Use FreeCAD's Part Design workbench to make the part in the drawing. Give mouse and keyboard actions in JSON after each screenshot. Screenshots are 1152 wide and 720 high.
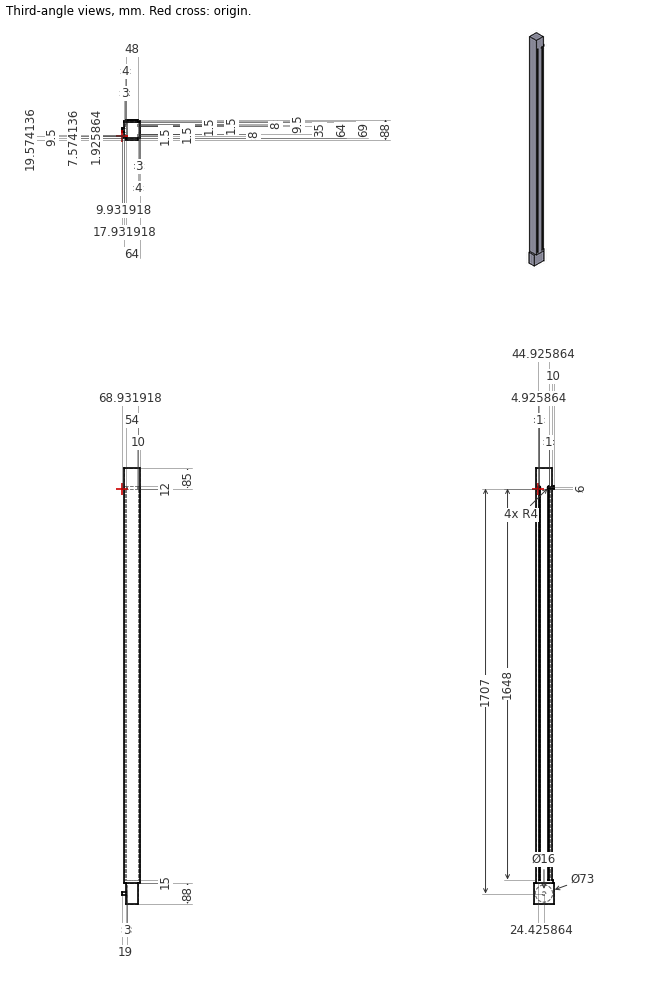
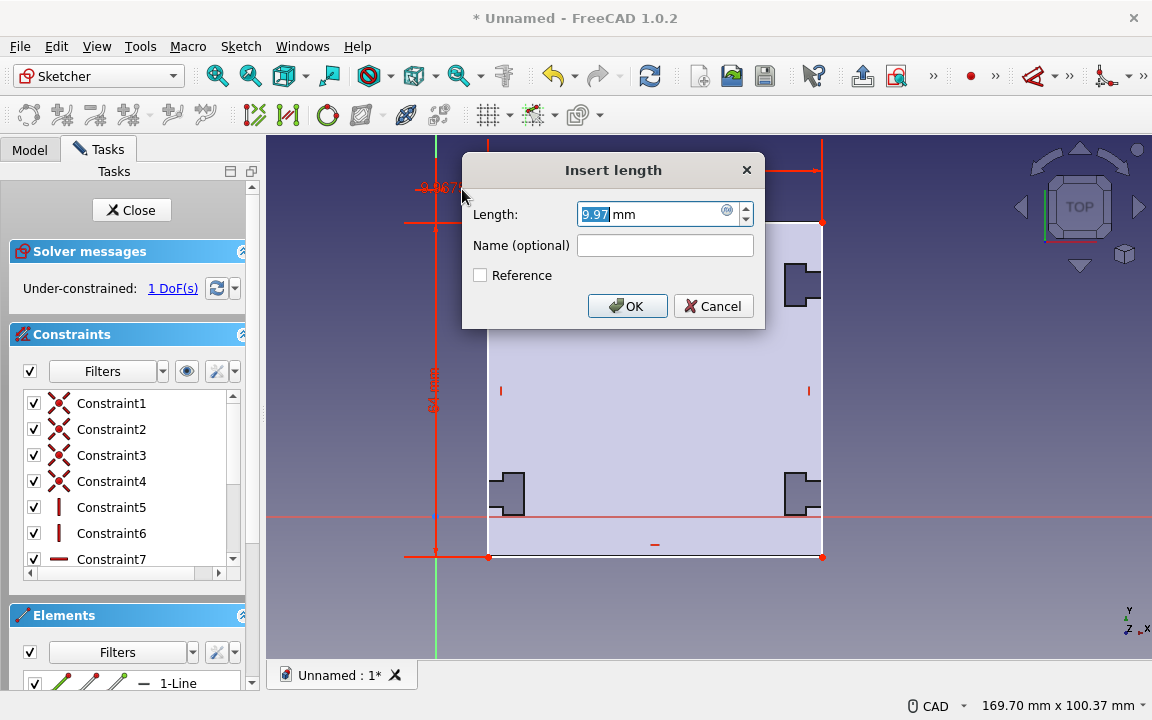
{"action": "type", "text": "9.931918"}
{"action": "key", "text": "Return"}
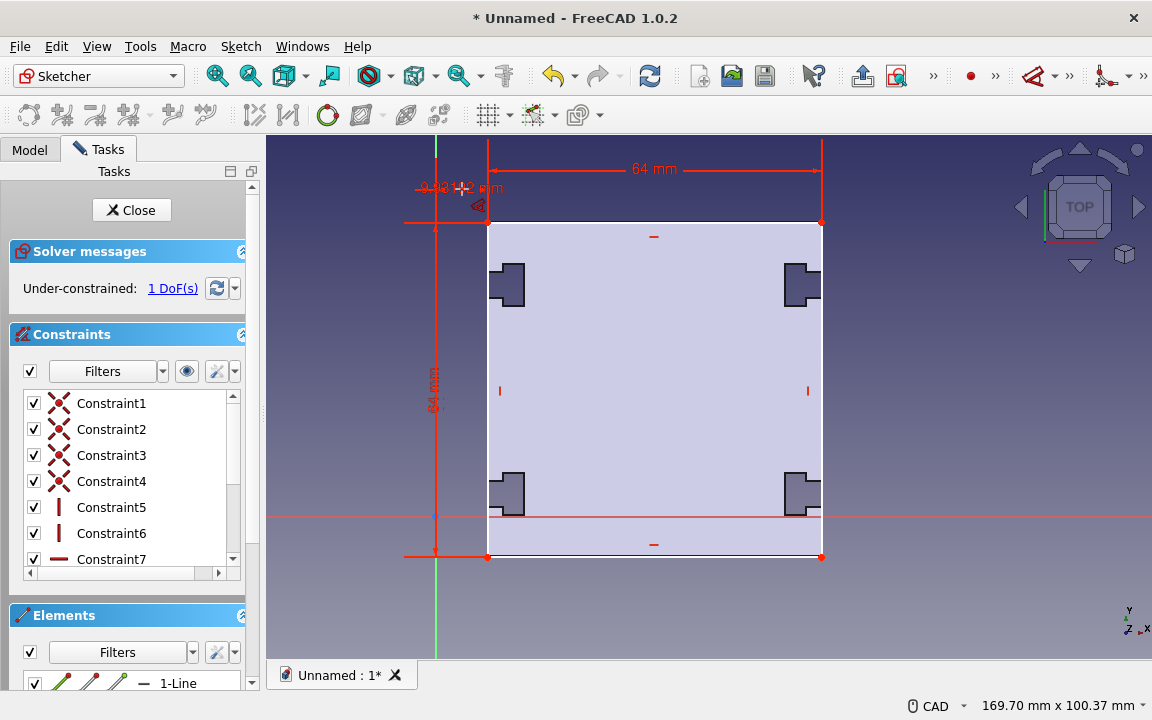
{"action": "left_click", "coordinate": [488, 557]}
{"action": "left_click", "coordinate": [402, 537]}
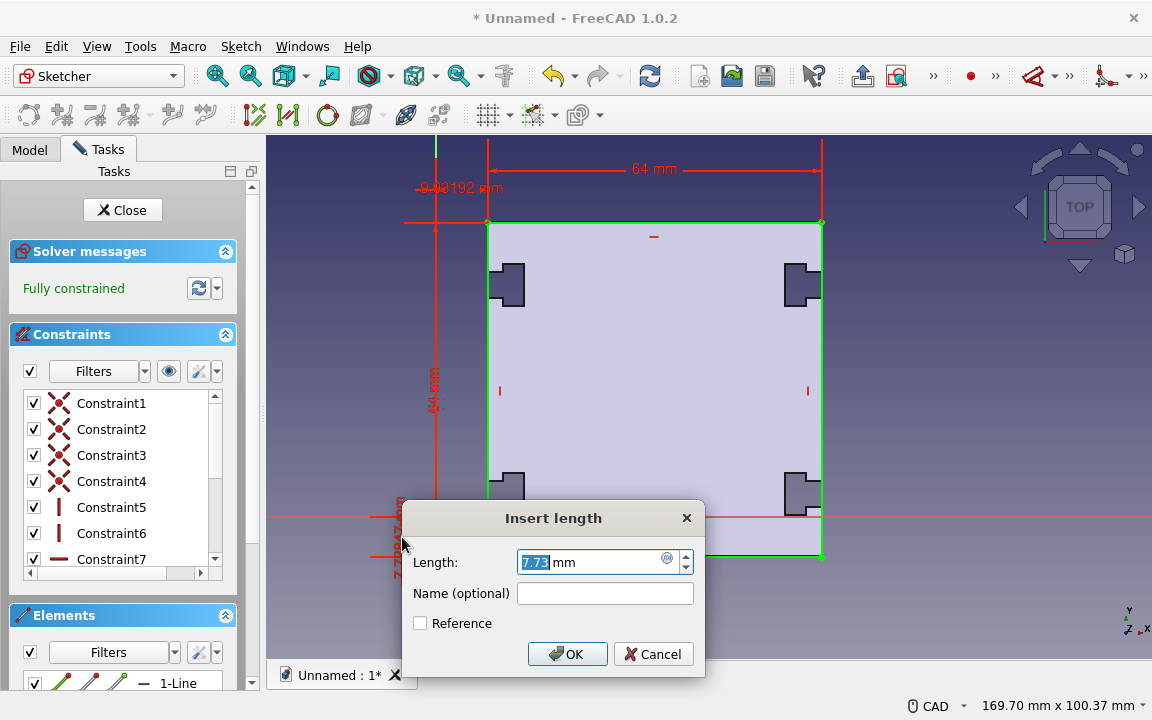
{"action": "type", "text": "7.574136"}
{"action": "key", "text": "Return"}
{"action": "key", "text": "Escape"}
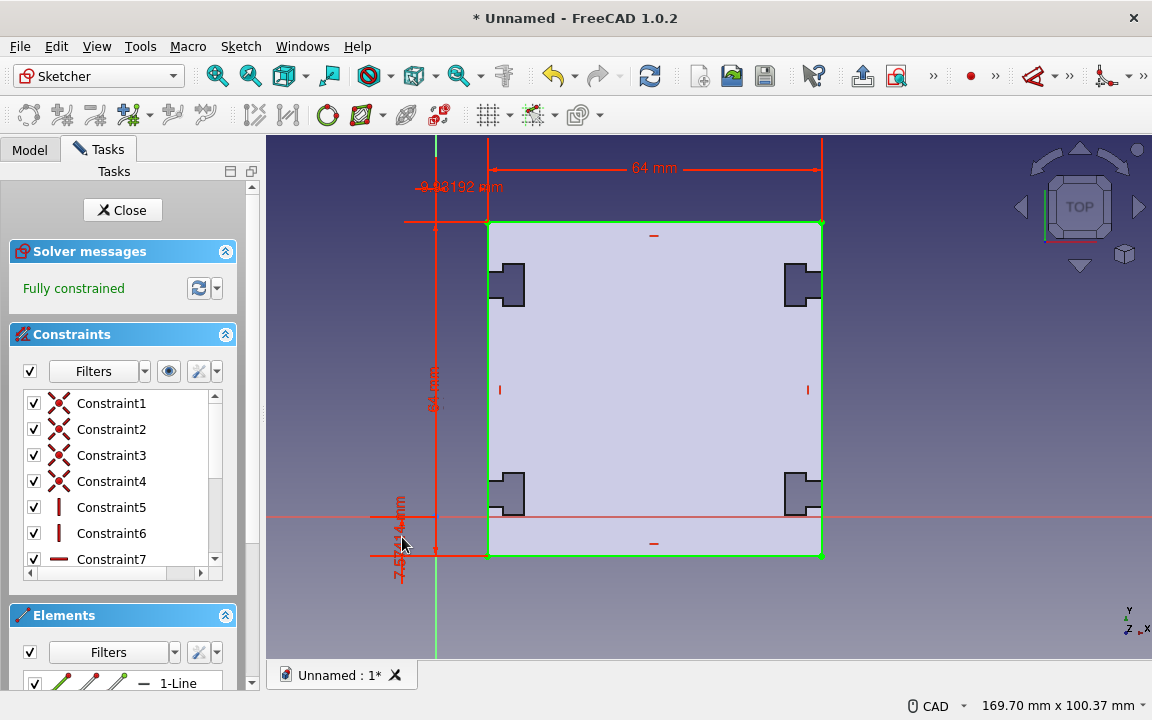
{"action": "left_click", "coordinate": [123, 210]}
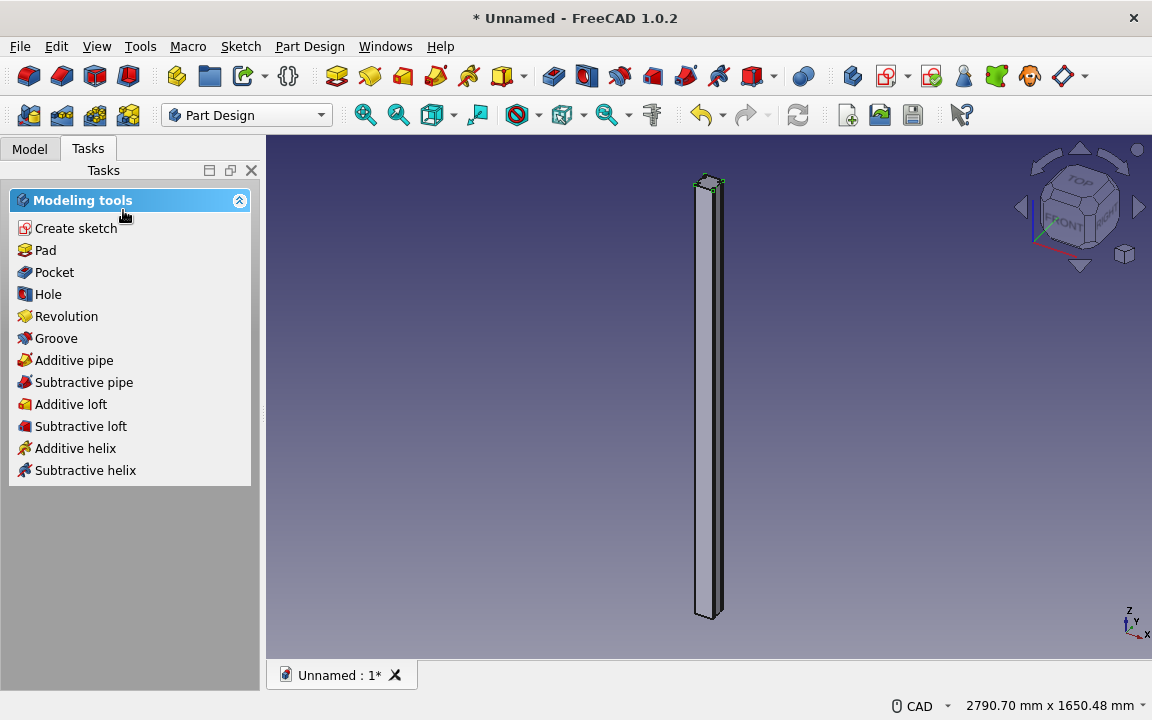
{"action": "left_click", "coordinate": [337, 76]}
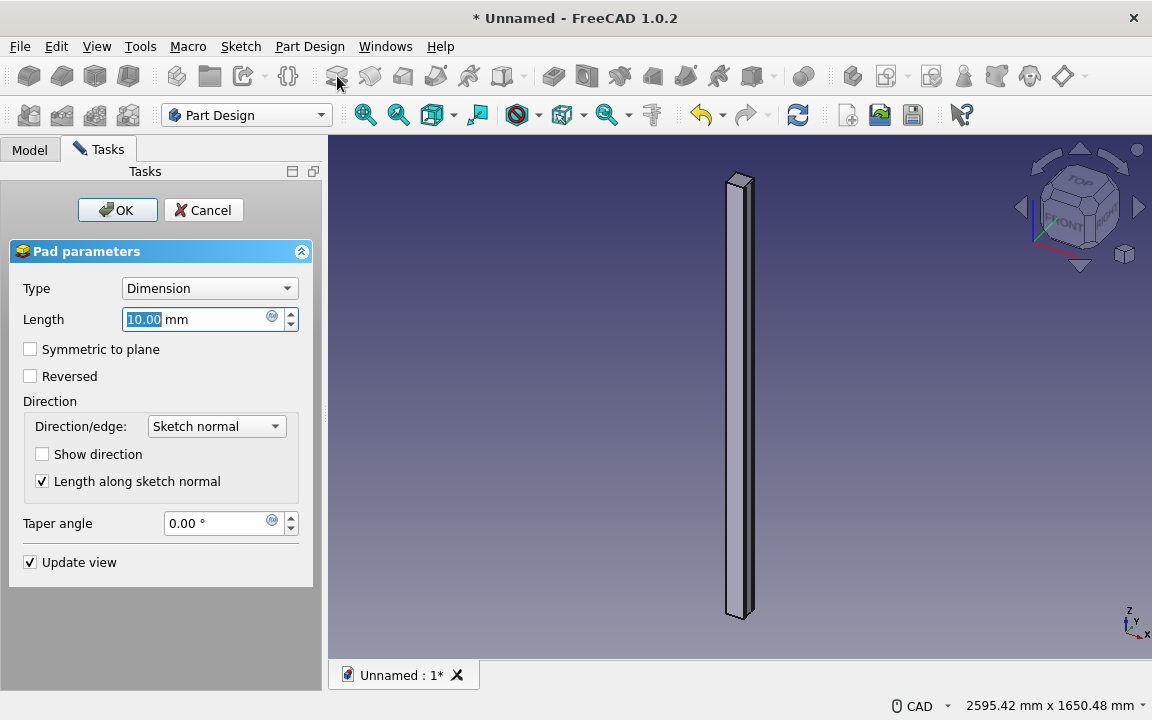
{"action": "type", "text": "85"}
{"action": "key", "text": "Tab"}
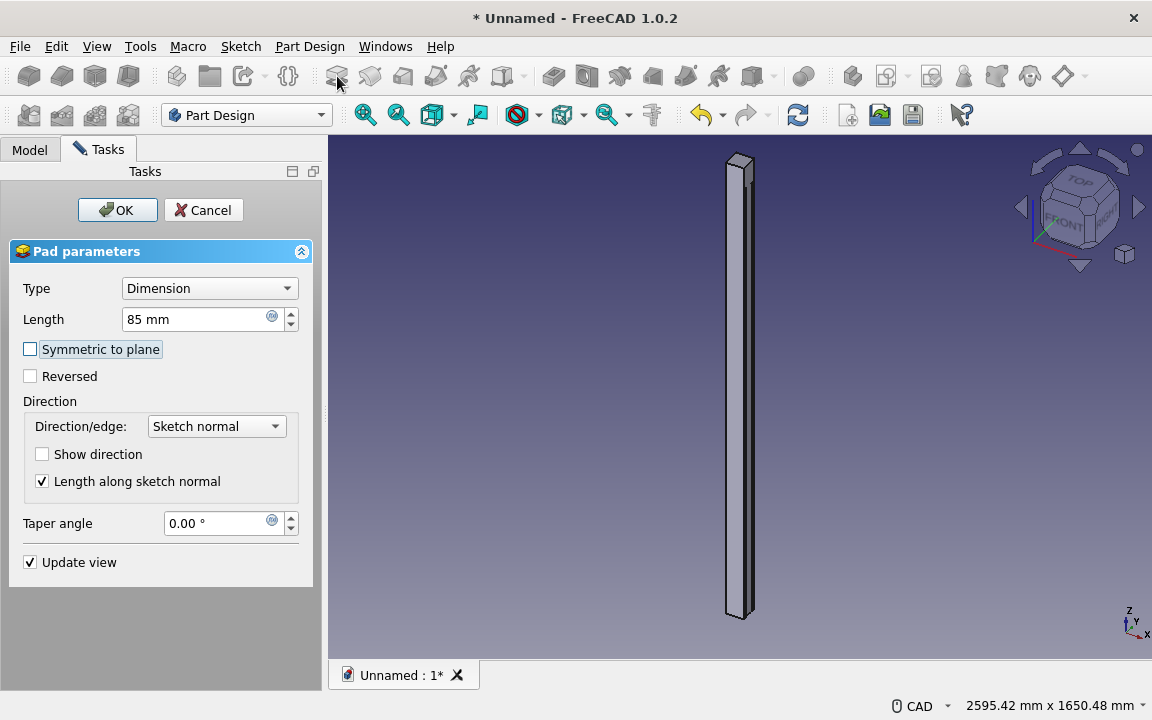
{"action": "left_click", "coordinate": [118, 210]}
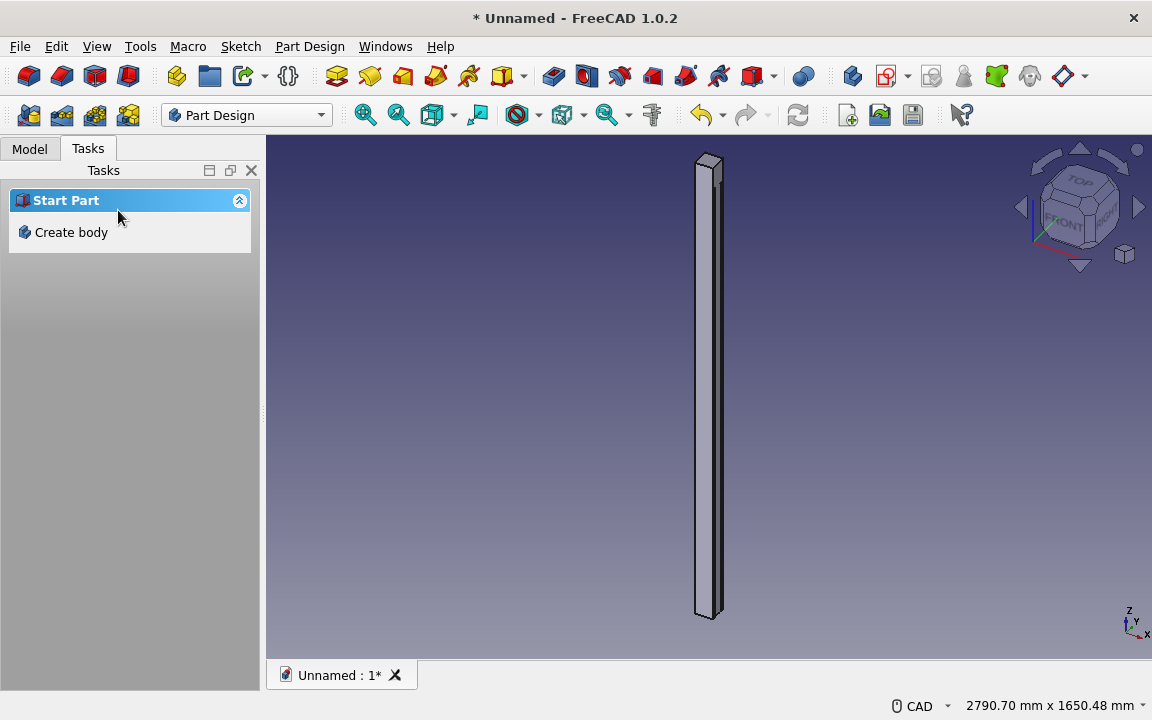
{"action": "key", "text": "4"}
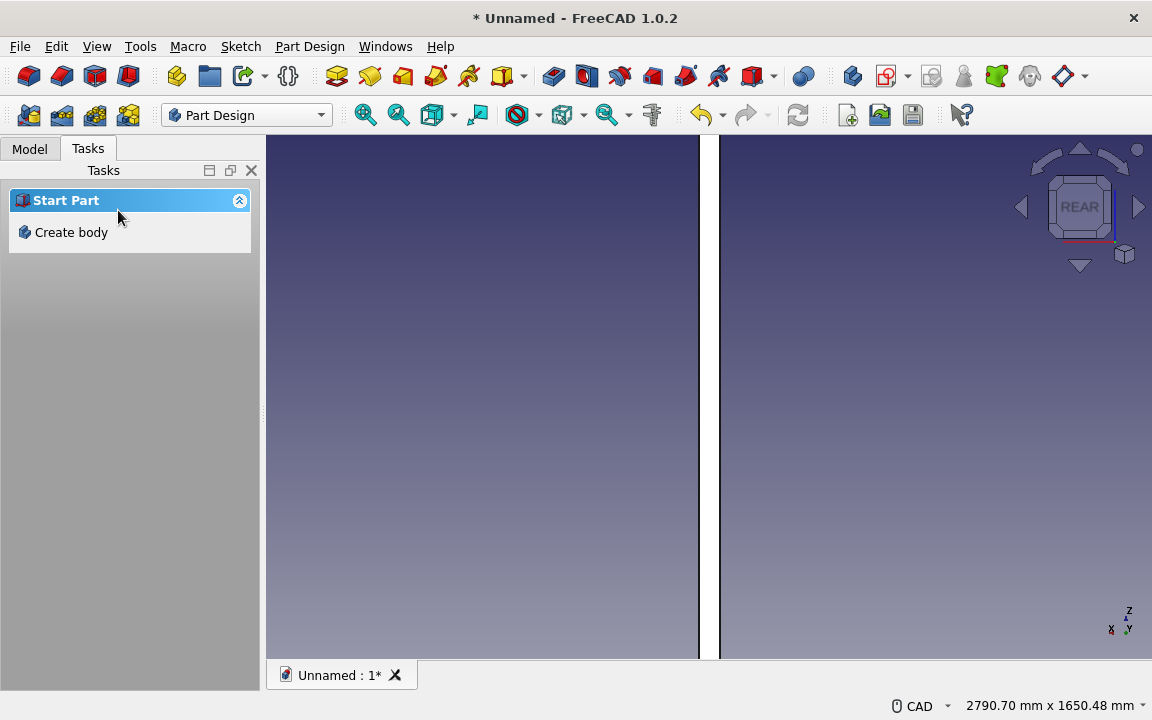
{"action": "left_click", "coordinate": [366, 116]}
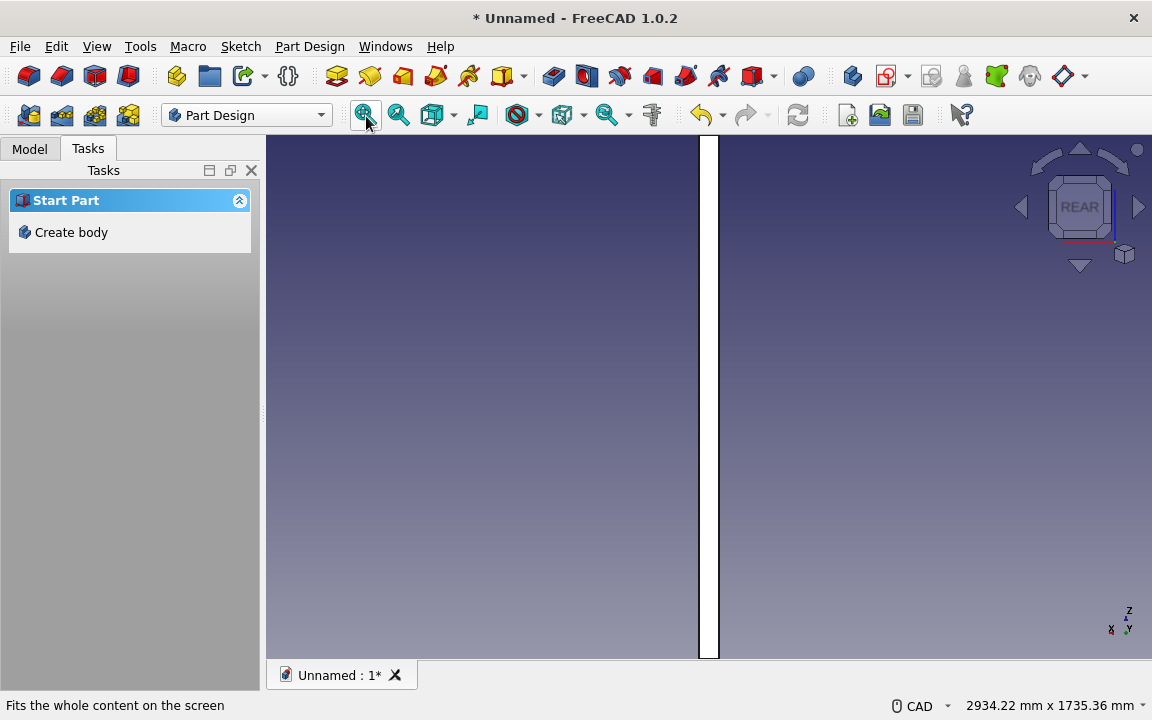
{"action": "left_click", "coordinate": [709, 172]}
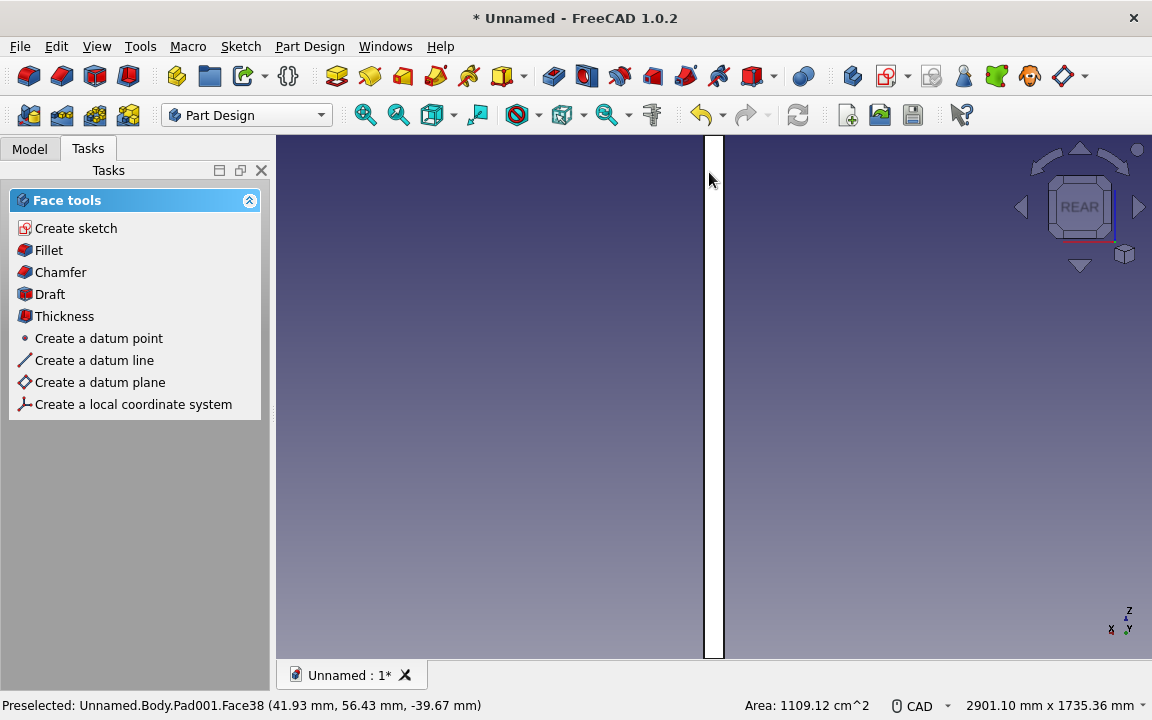
{"action": "left_click", "coordinate": [886, 76]}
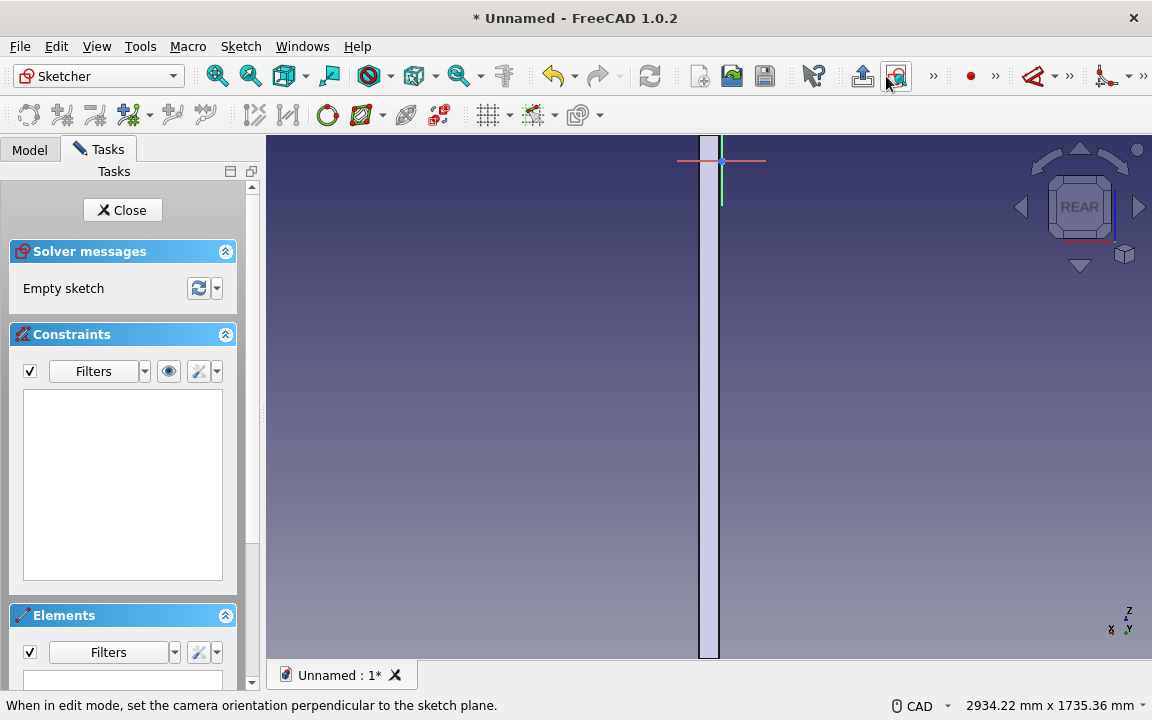
{"action": "scroll", "coordinate": [640, 397], "scroll_direction": "down", "scroll_amount": 5}